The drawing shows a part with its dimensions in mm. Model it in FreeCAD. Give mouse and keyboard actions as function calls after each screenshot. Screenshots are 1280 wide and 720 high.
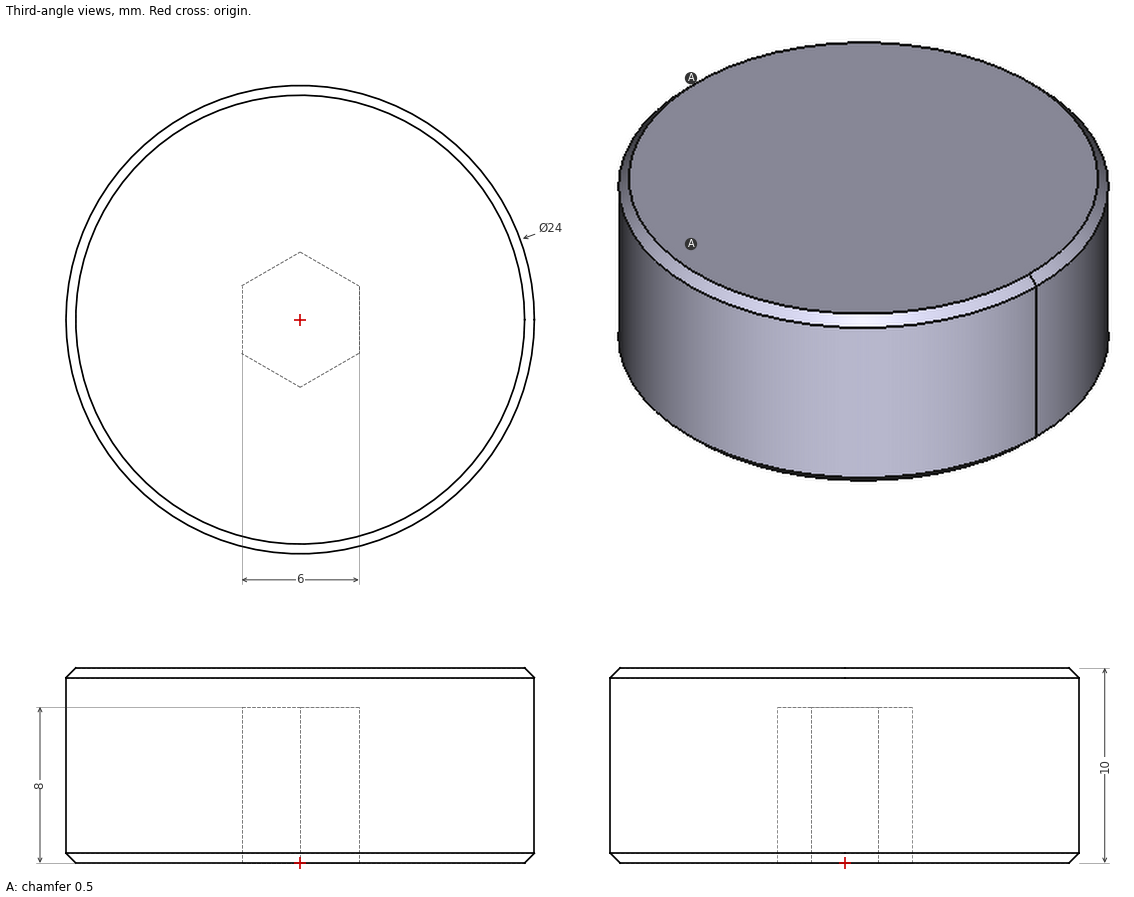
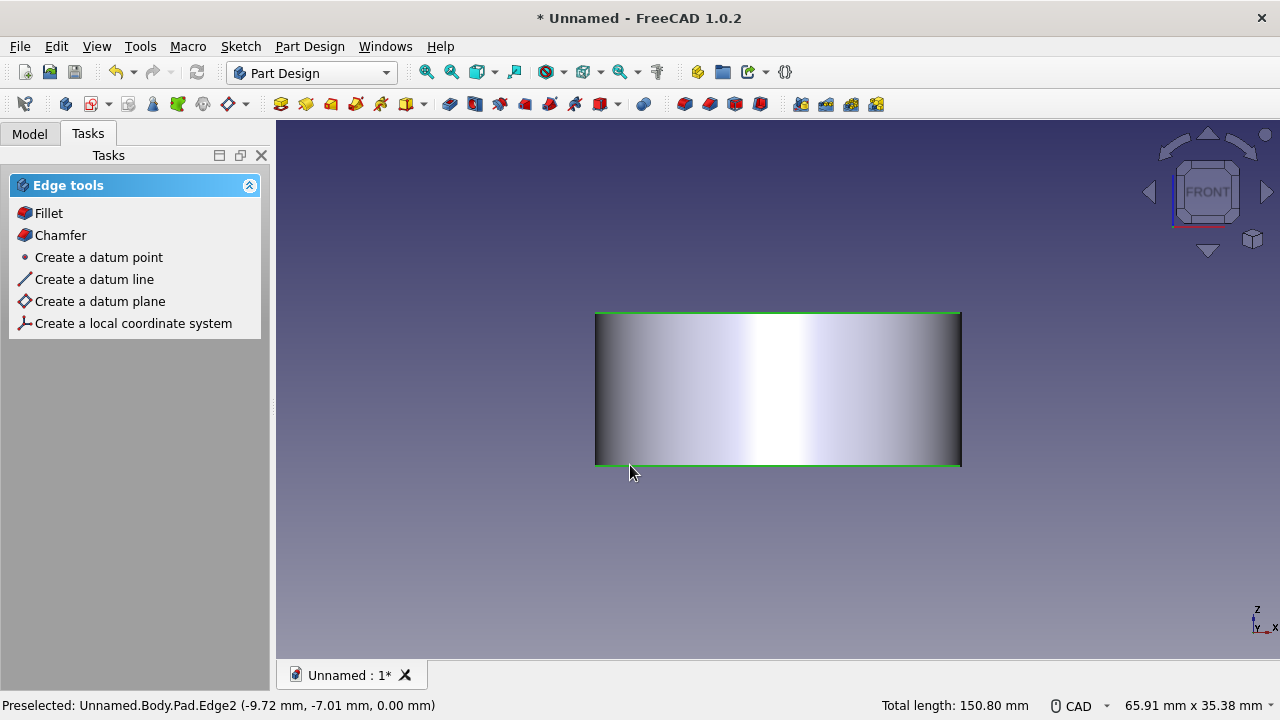
click(710, 104)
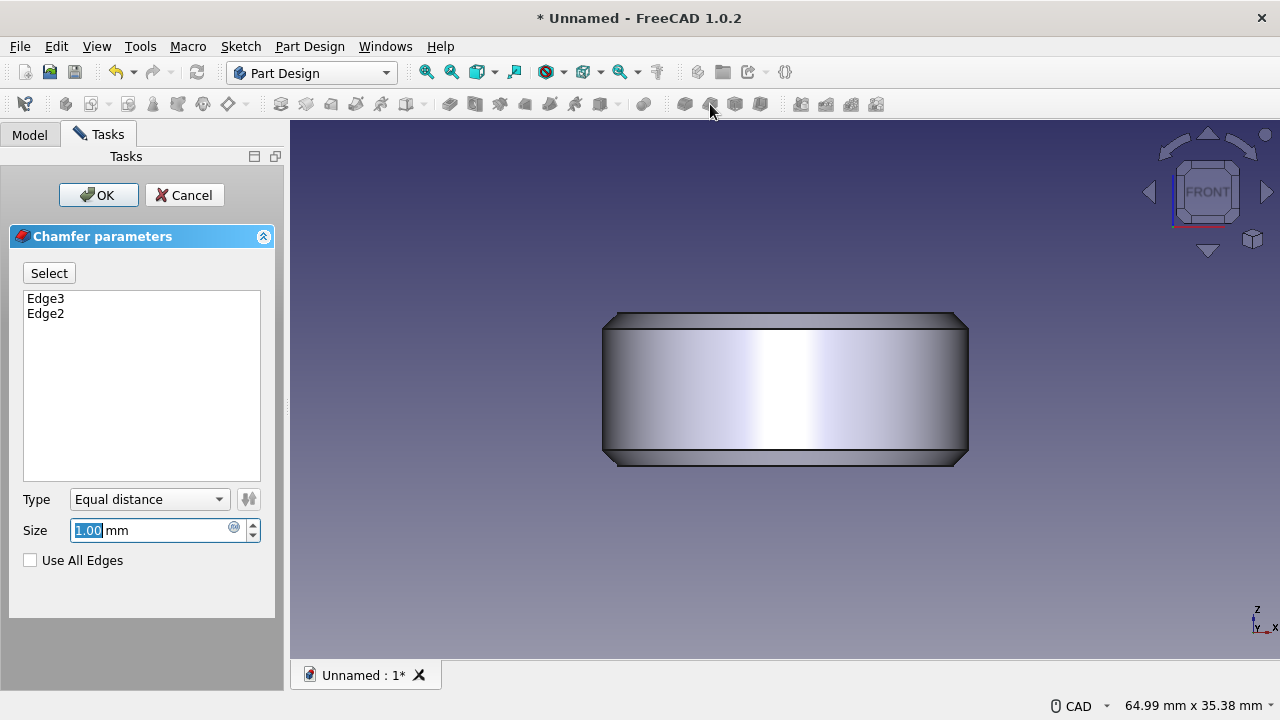
text(0.5)
key(Tab)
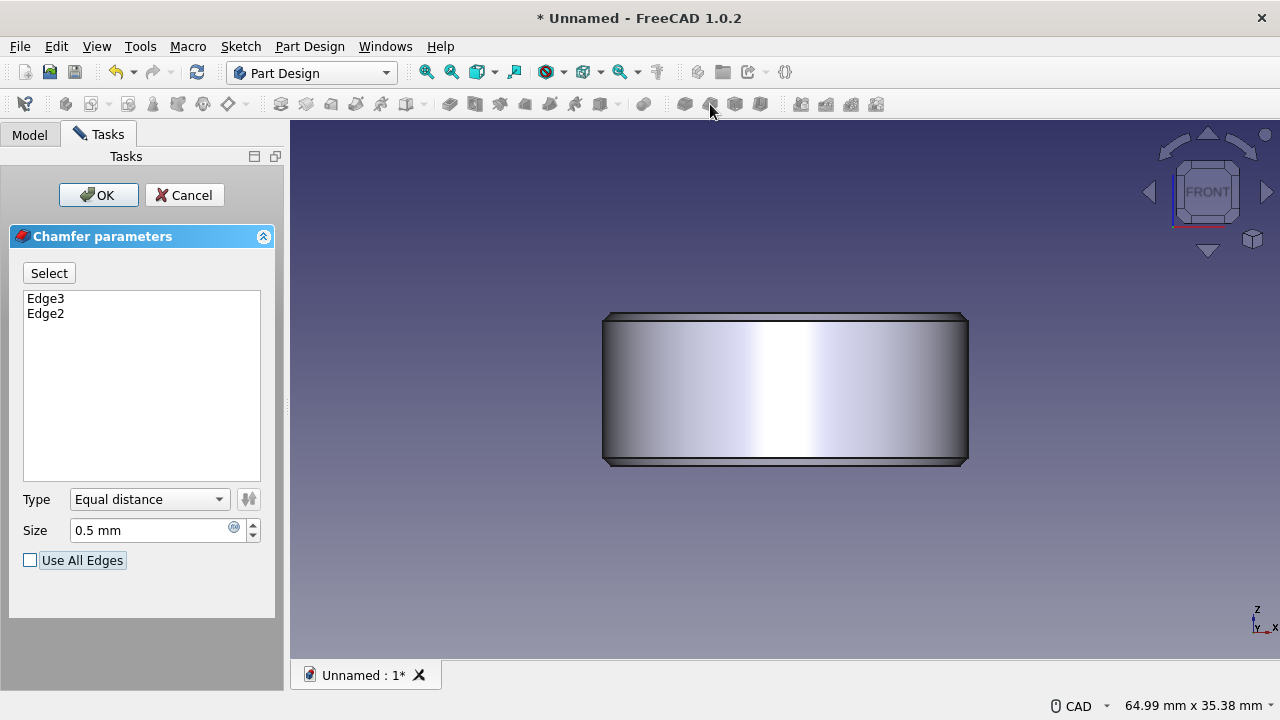
click(99, 195)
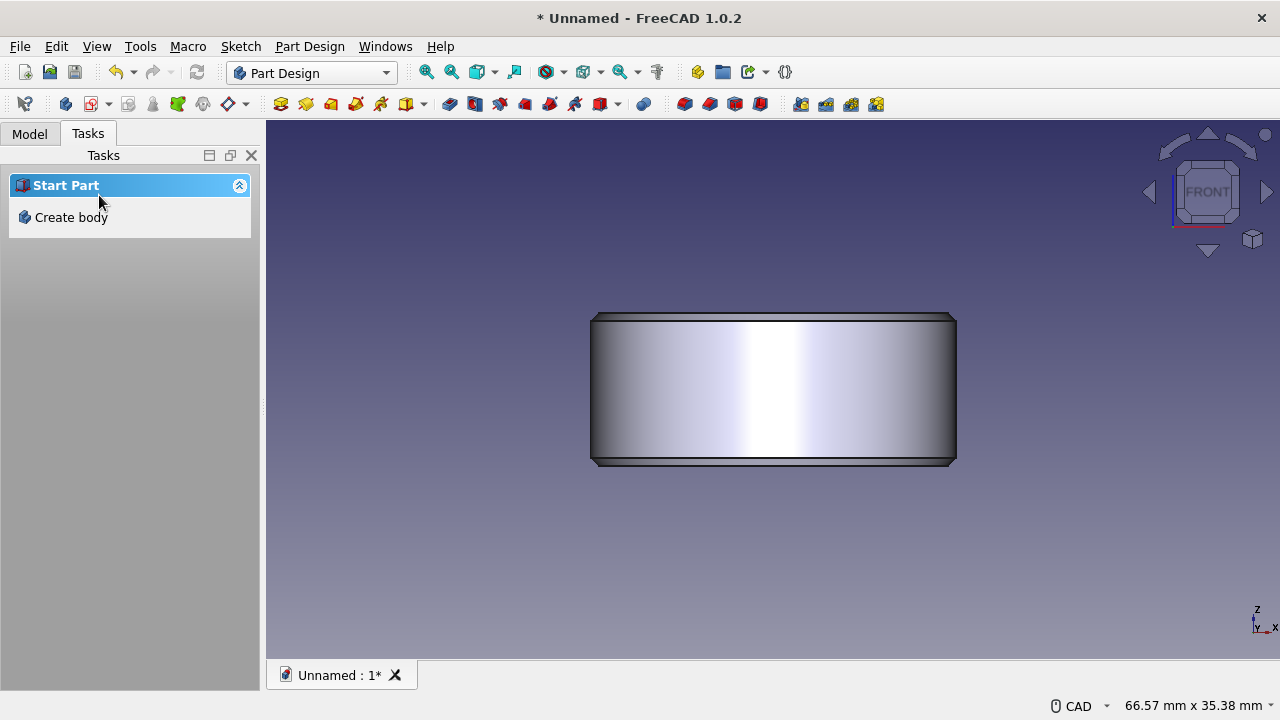
click(427, 72)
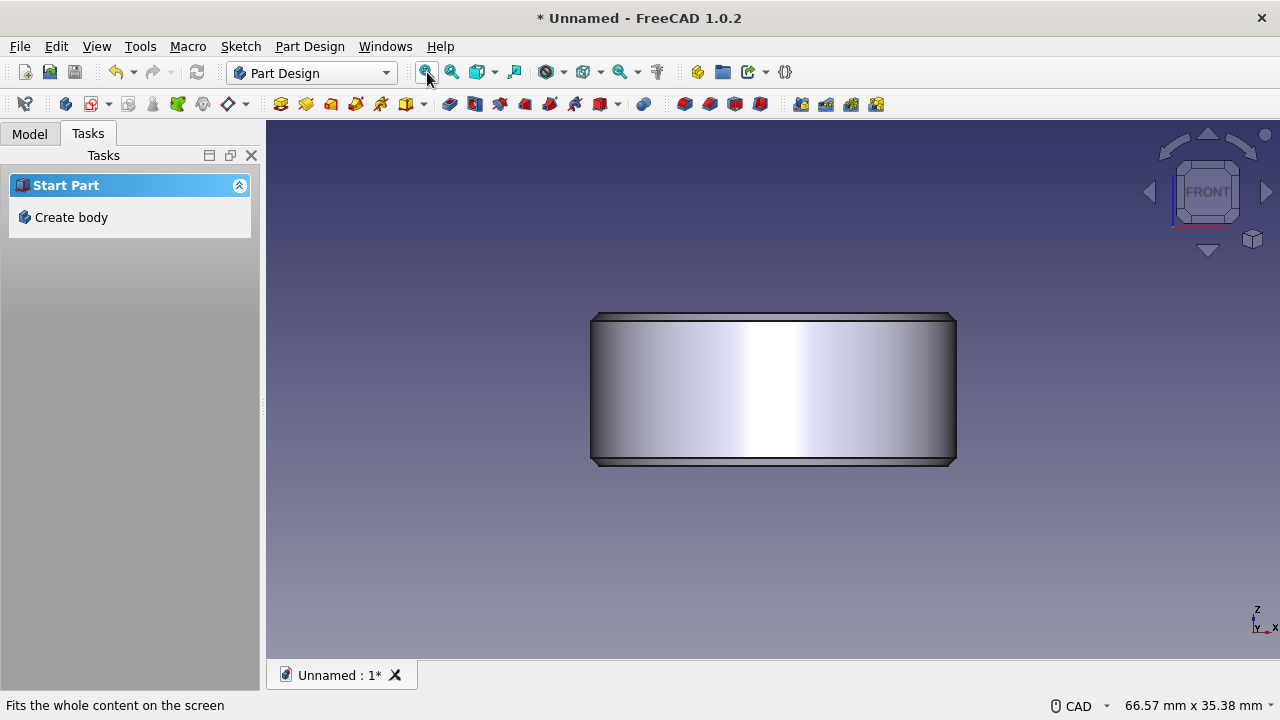
key(5)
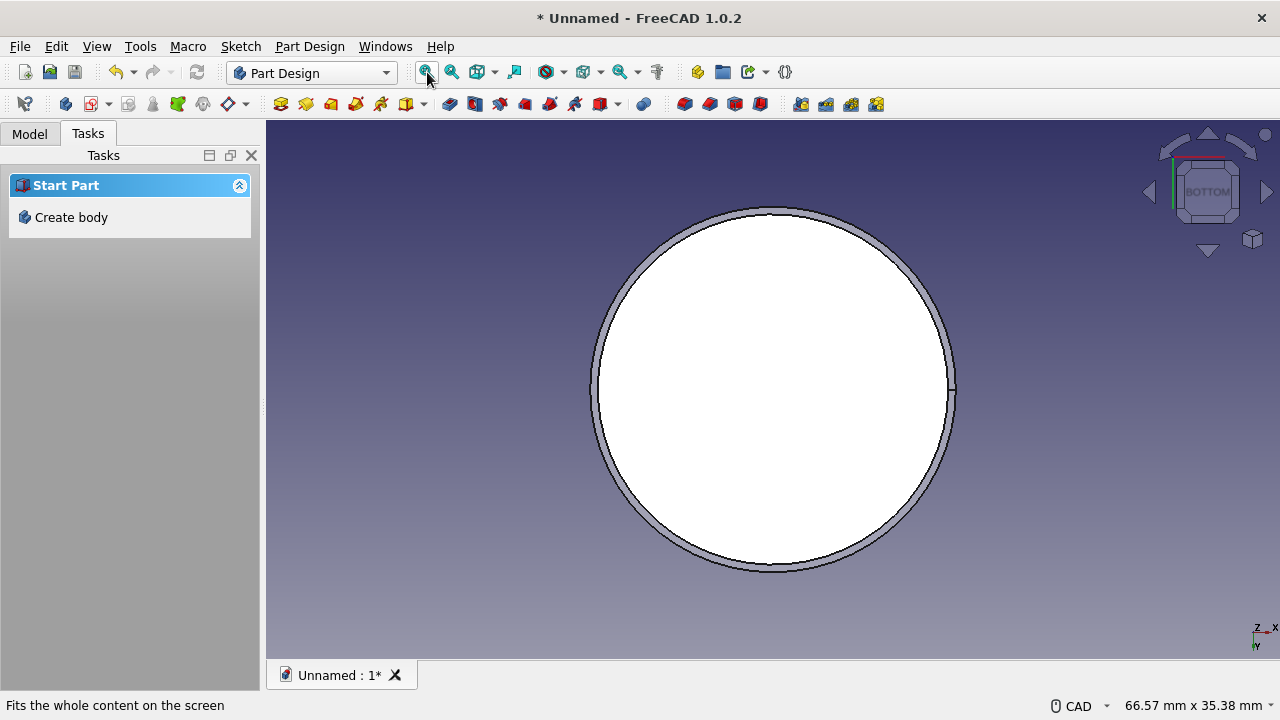
click(773, 388)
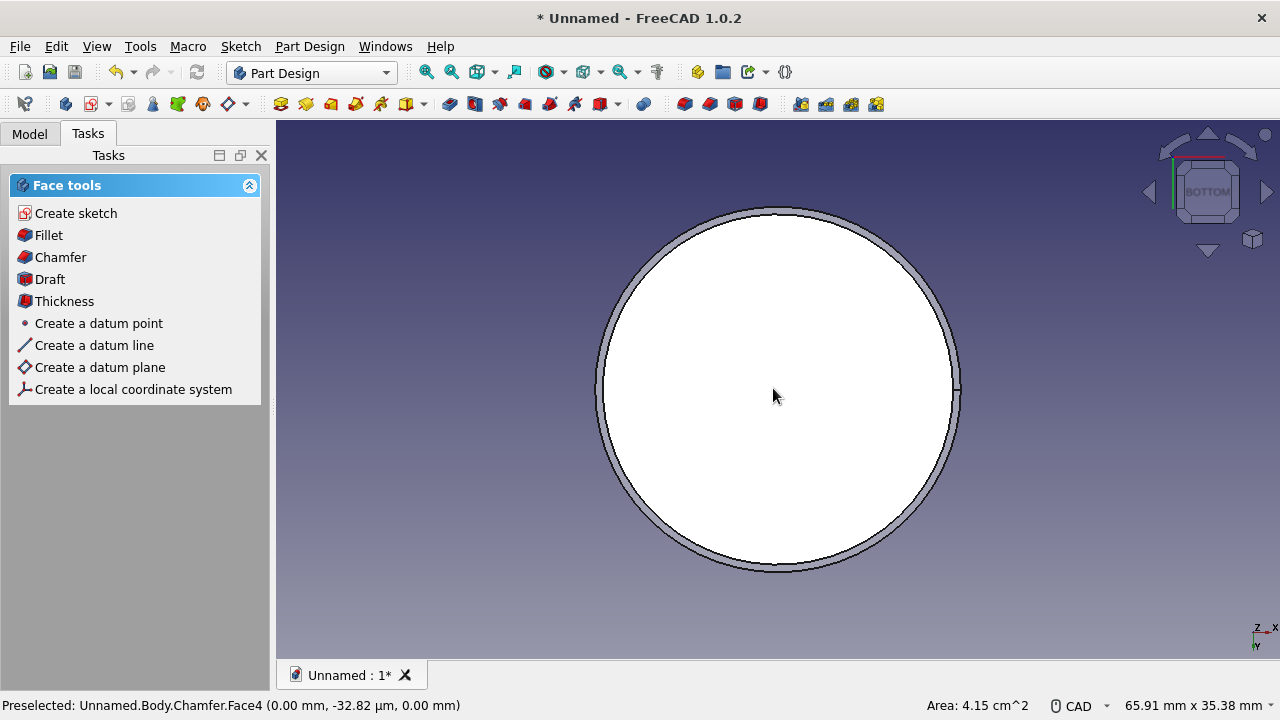
click(90, 104)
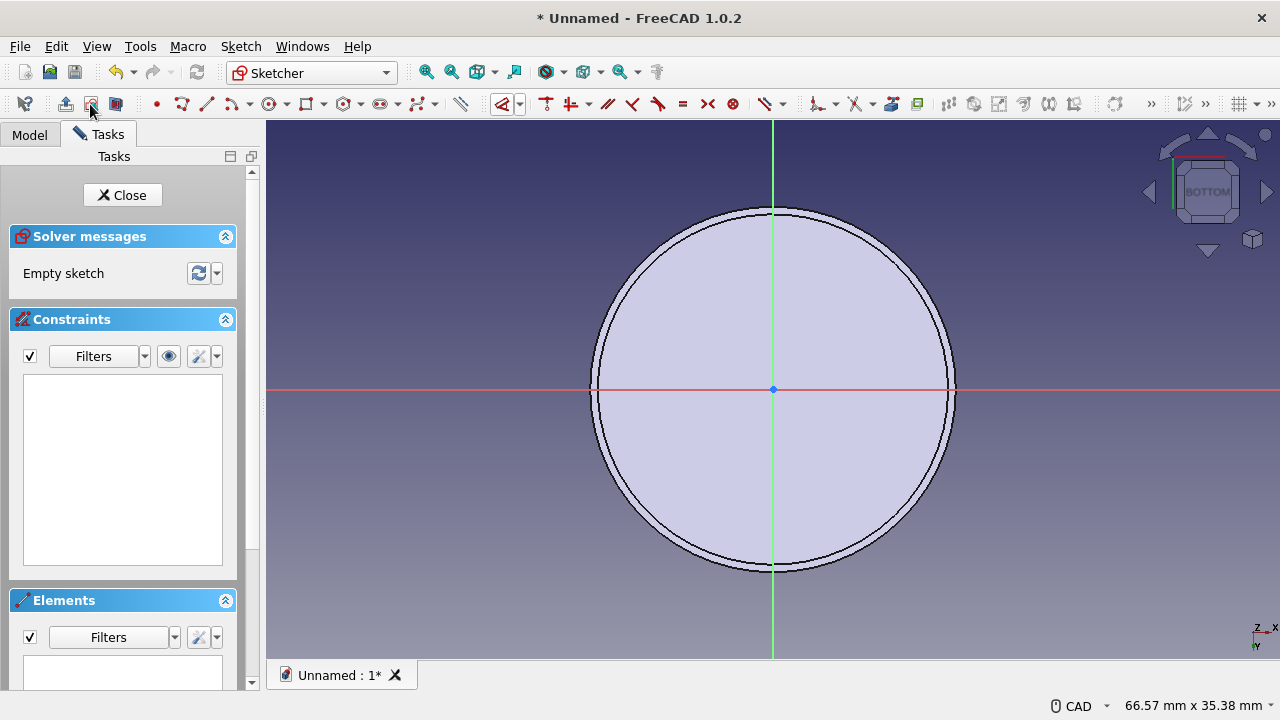
scroll(803, 390, up, 6)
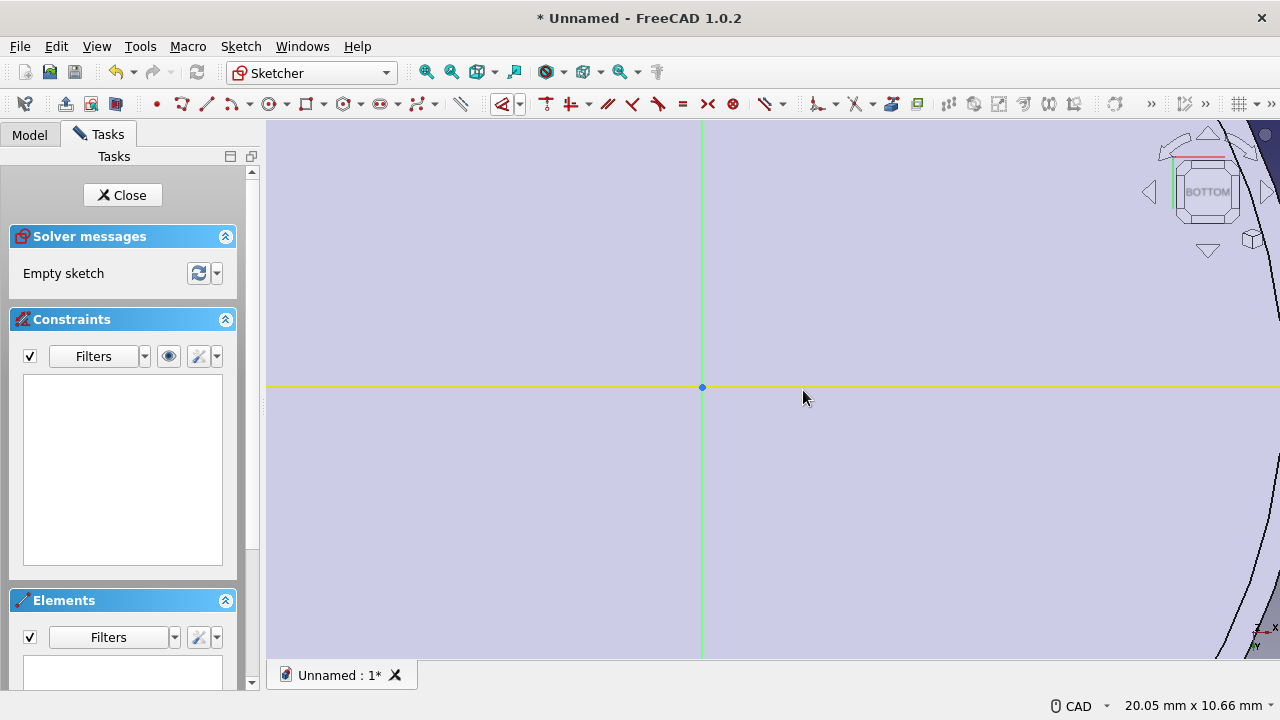
click(342, 104)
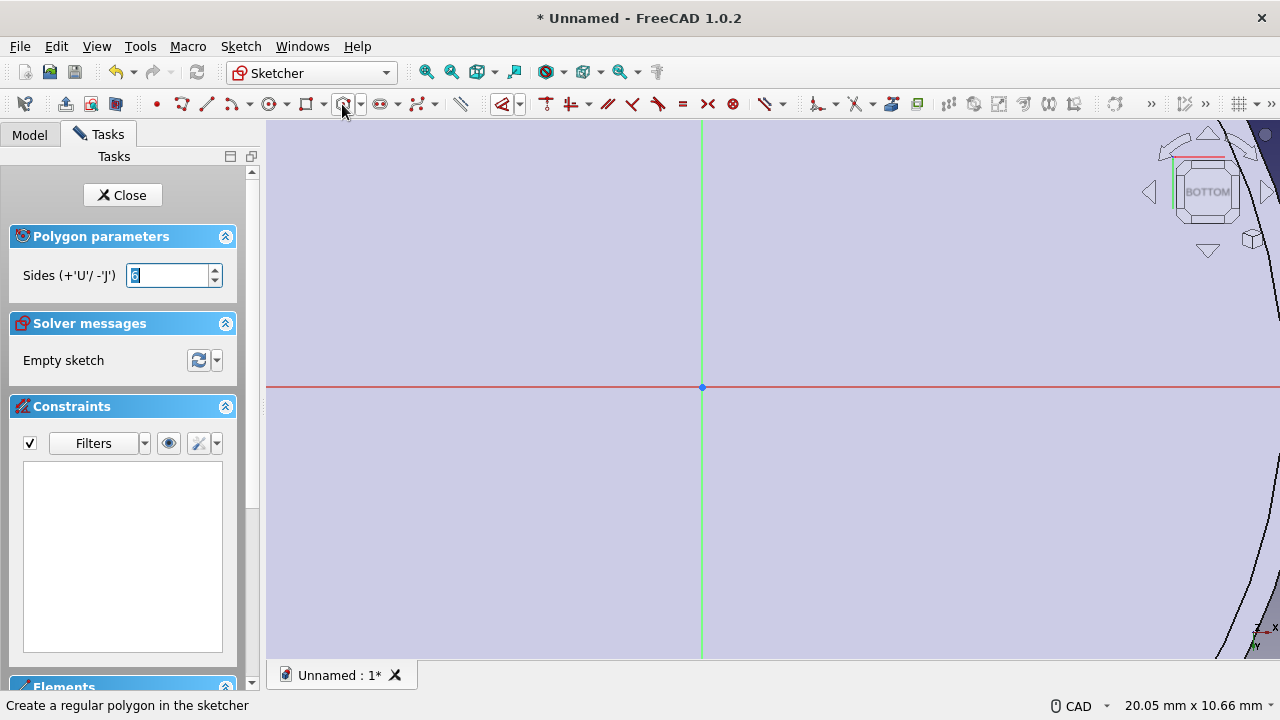
click(702, 387)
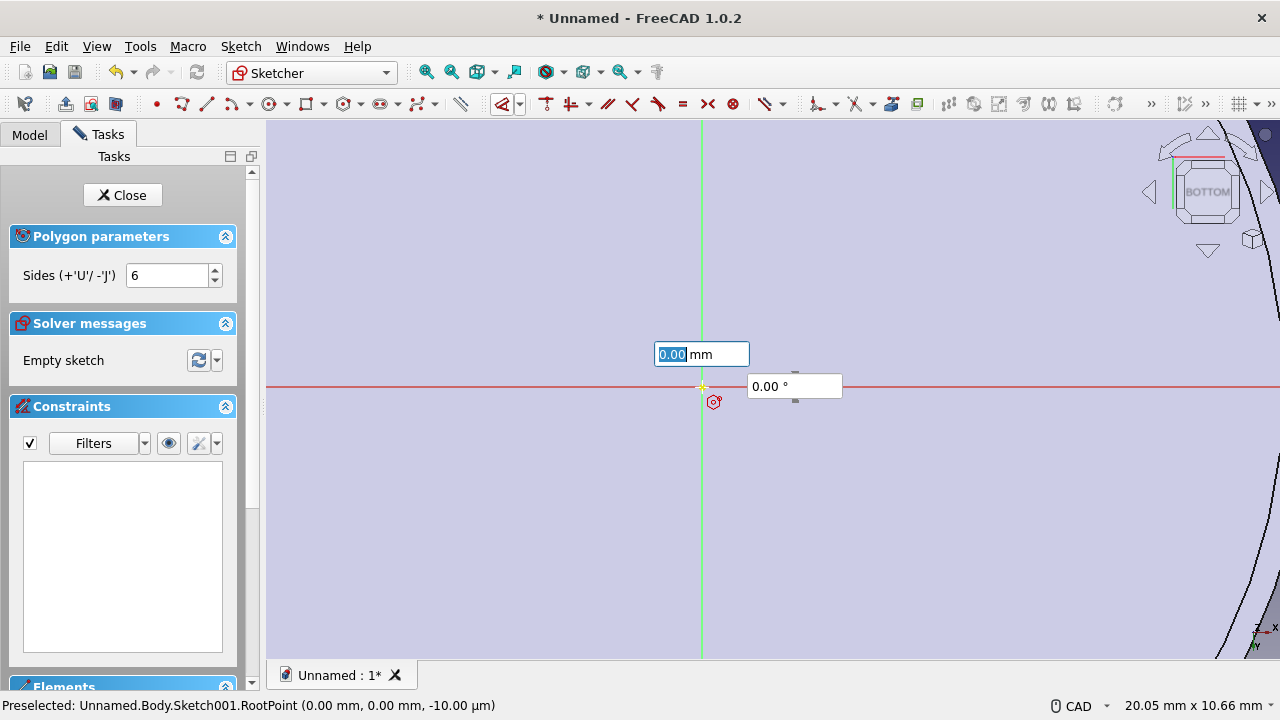
click(702, 212)
right_click(702, 212)